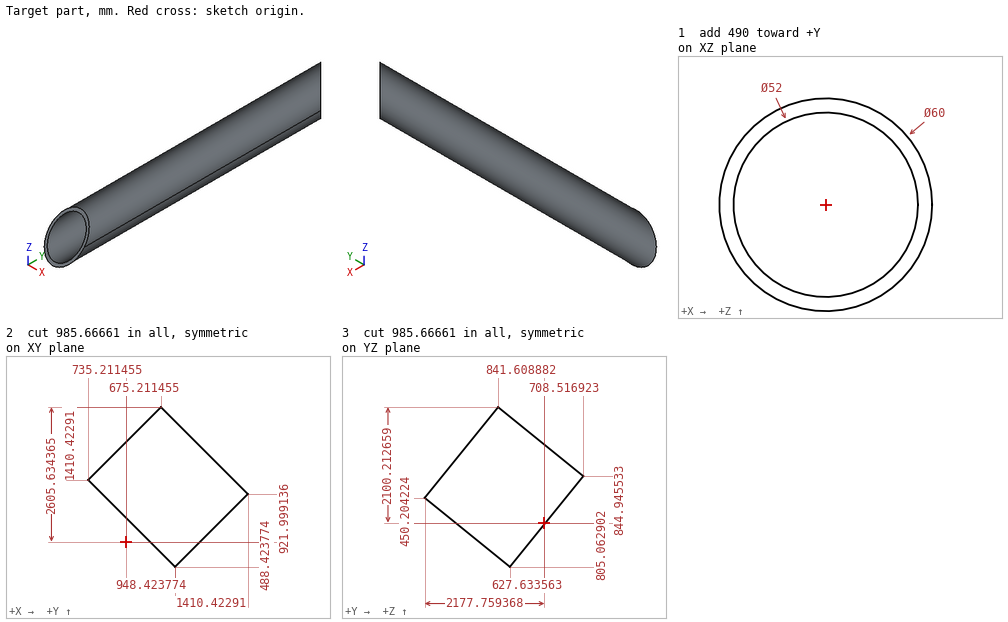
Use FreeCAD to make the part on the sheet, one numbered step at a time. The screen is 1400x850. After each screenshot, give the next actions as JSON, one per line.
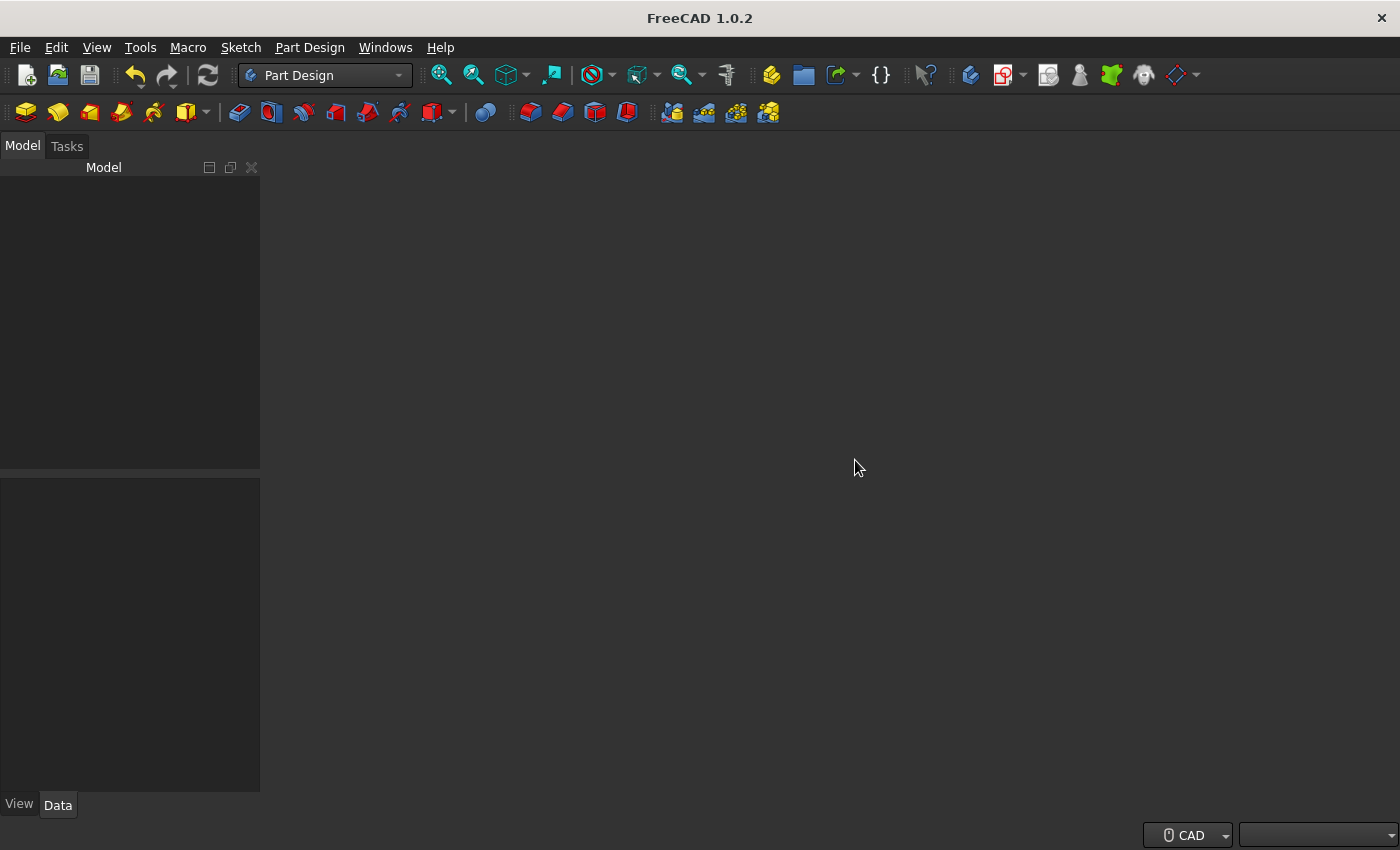
{"action": "key", "text": "ctrl+n"}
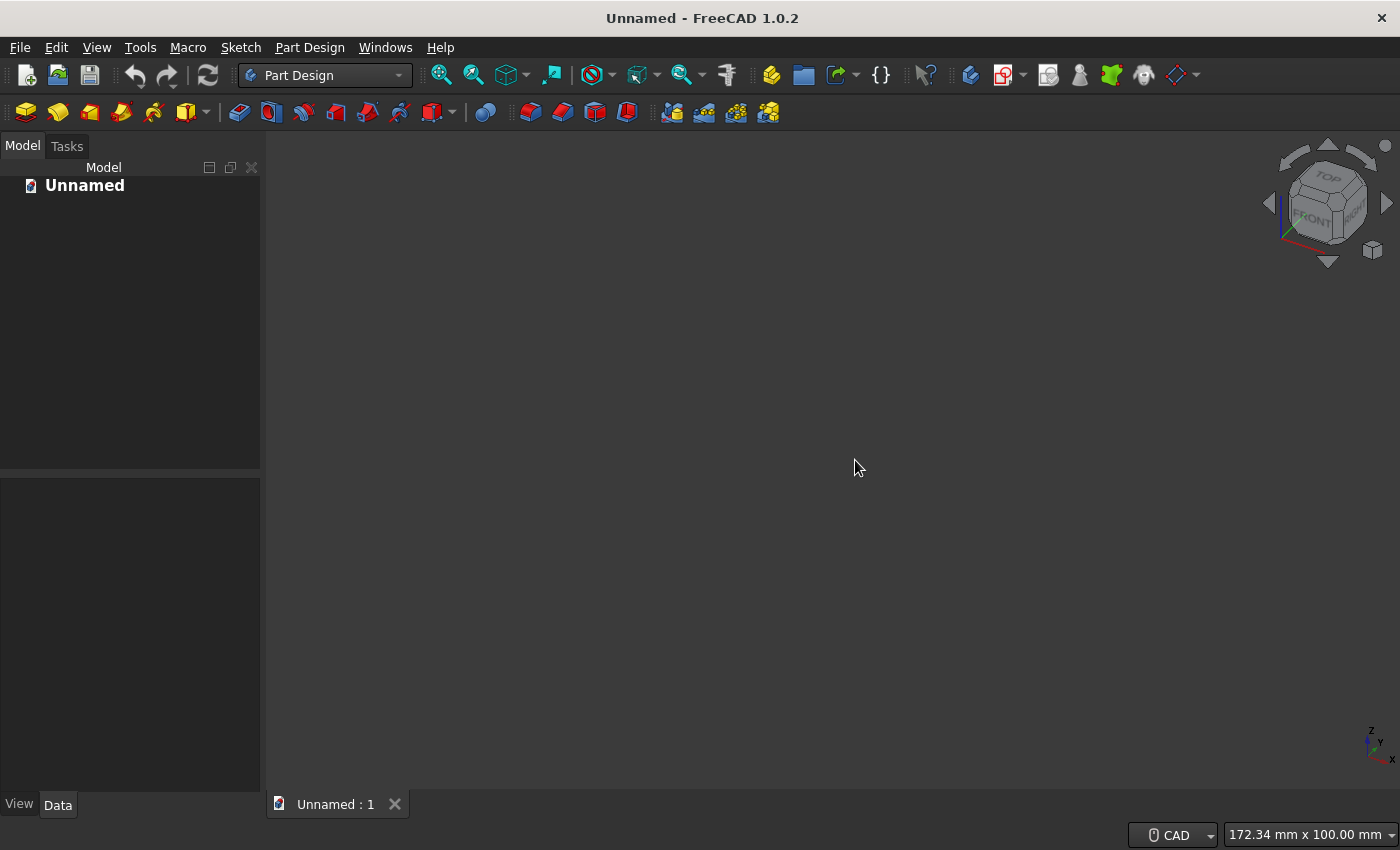
{"action": "left_click", "coordinate": [1004, 76]}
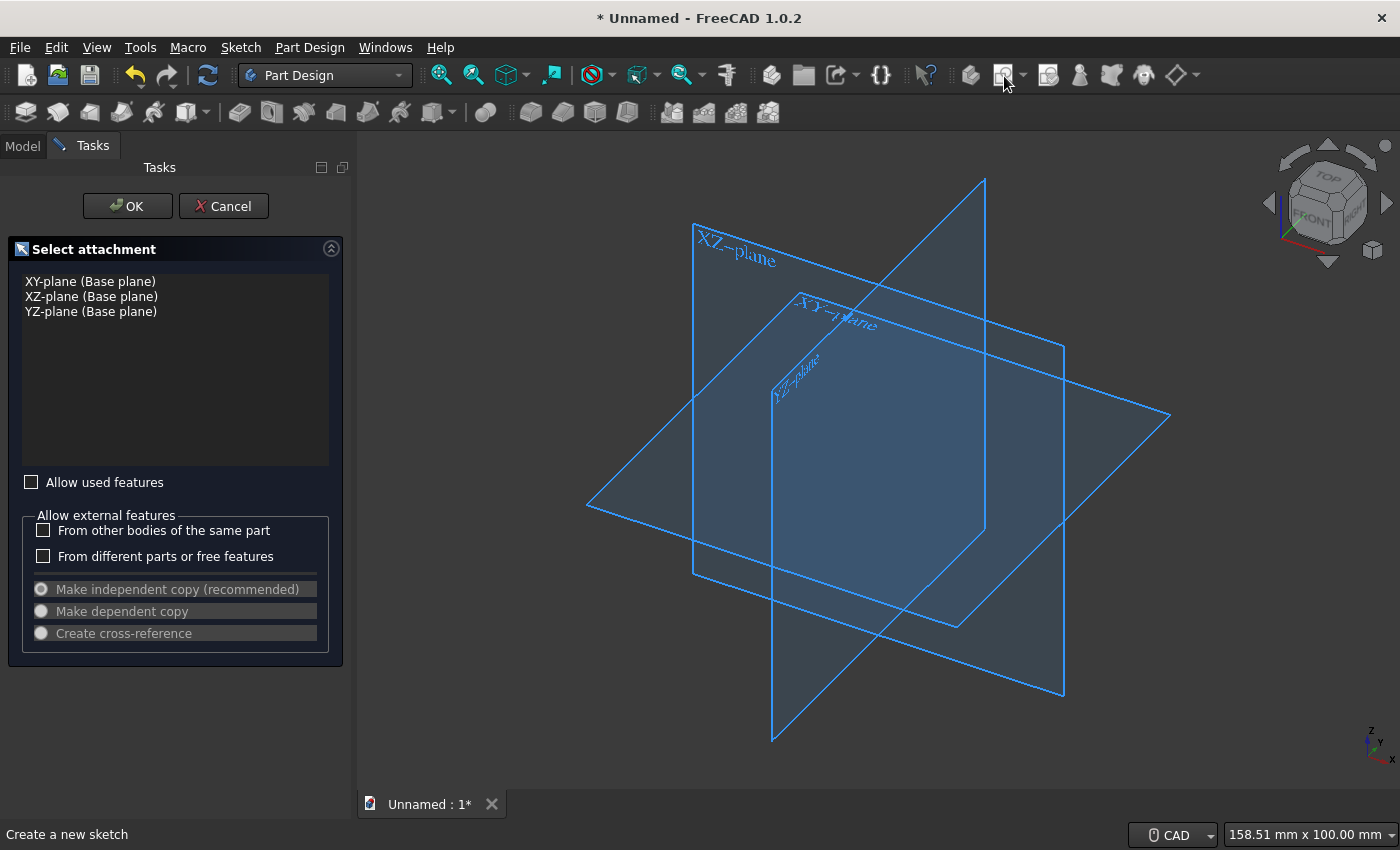
{"action": "left_click", "coordinate": [82, 296]}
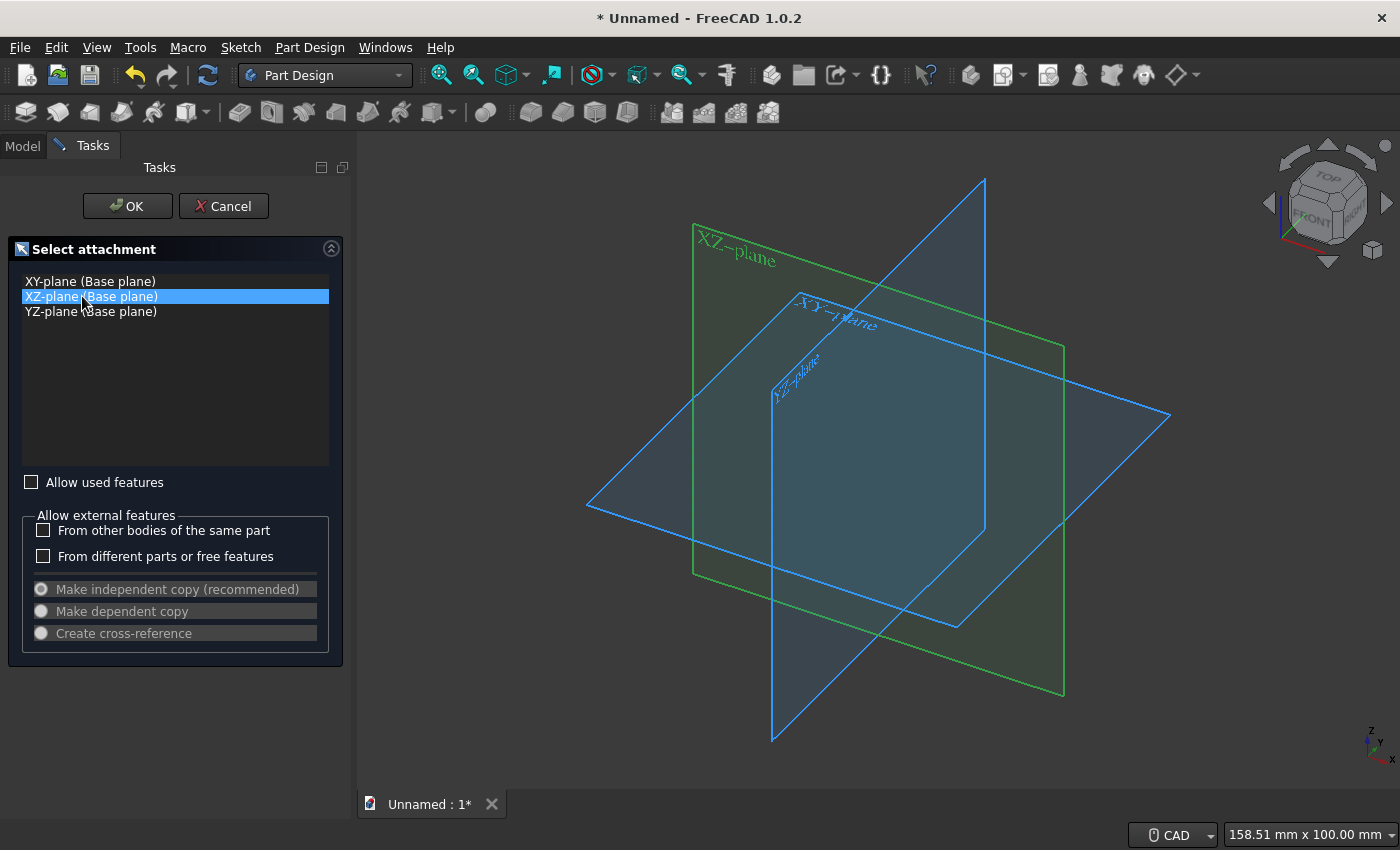
{"action": "left_click", "coordinate": [128, 206]}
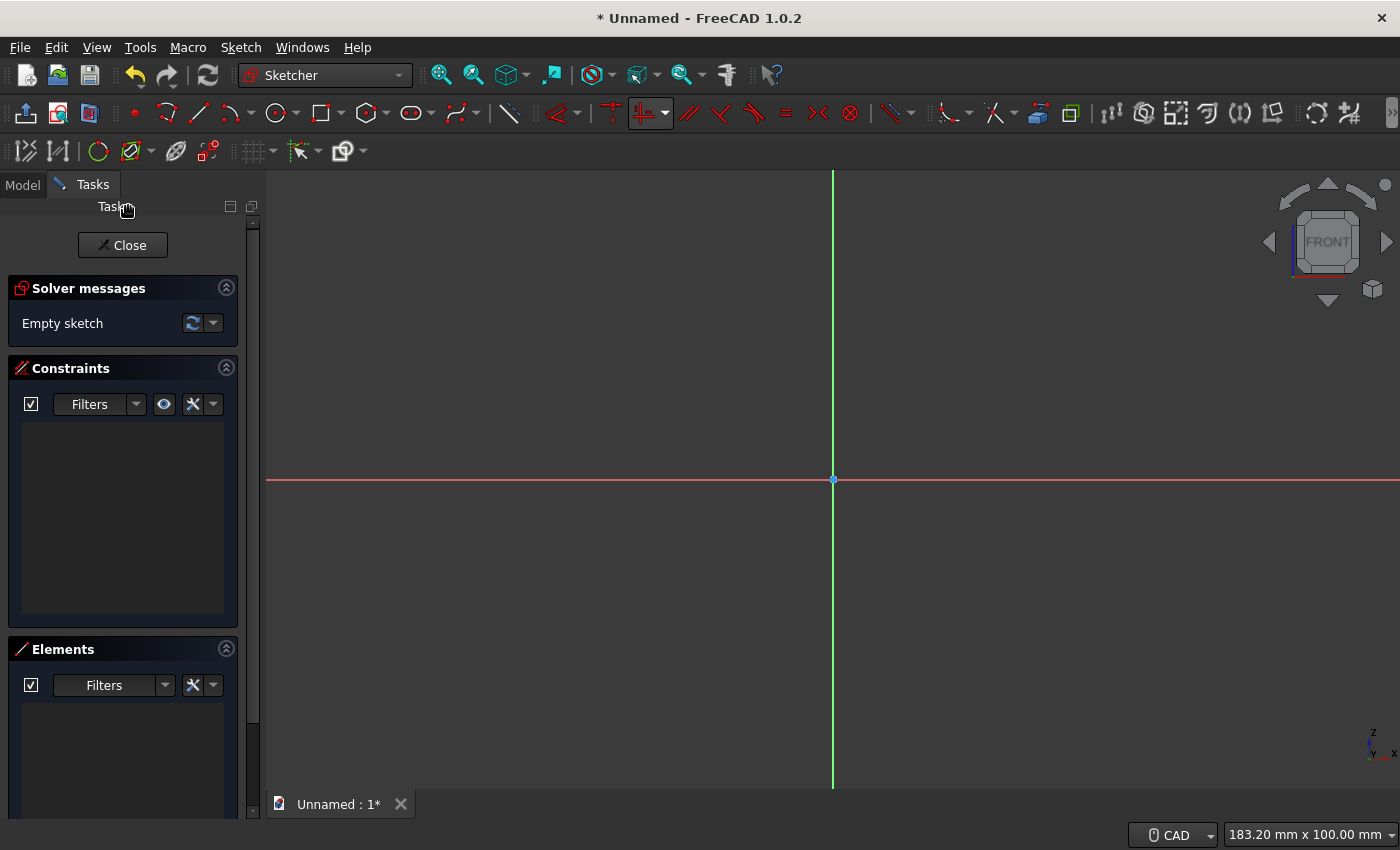
{"action": "key", "text": "g c"}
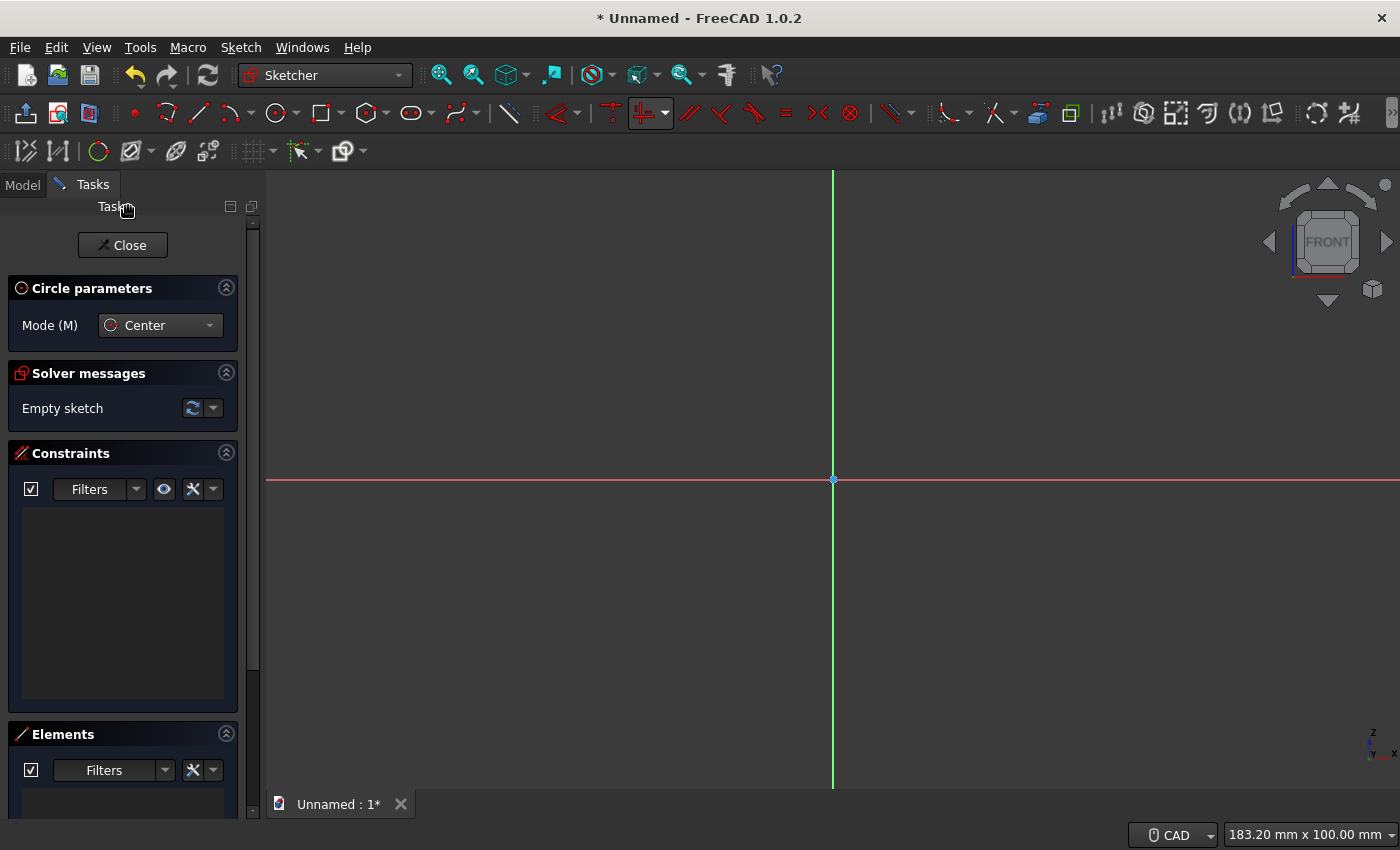
{"action": "left_click", "coordinate": [833, 480]}
{"action": "mouse_move", "coordinate": [964, 348]}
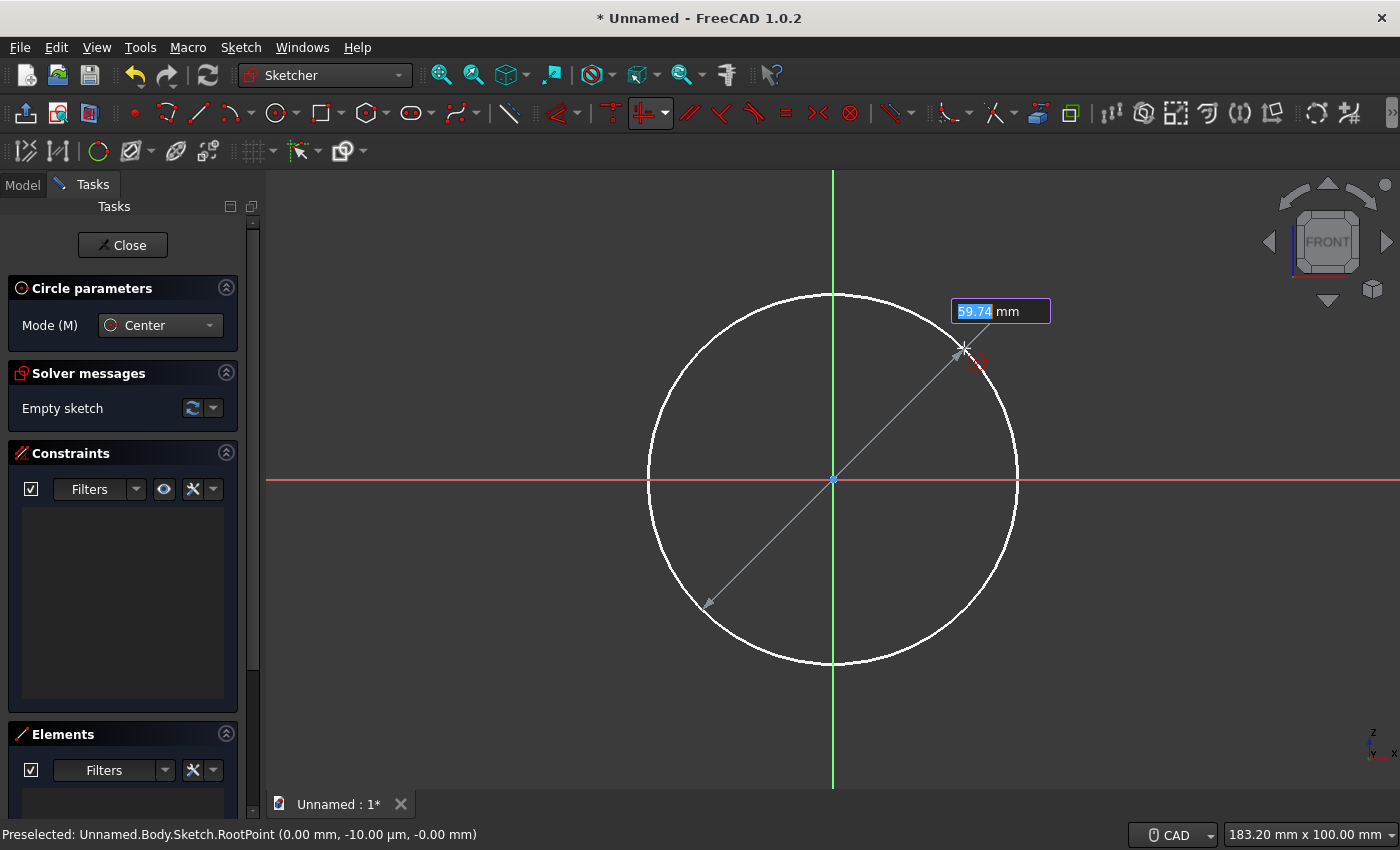
{"action": "type", "text": "60"}
{"action": "key", "text": "Return"}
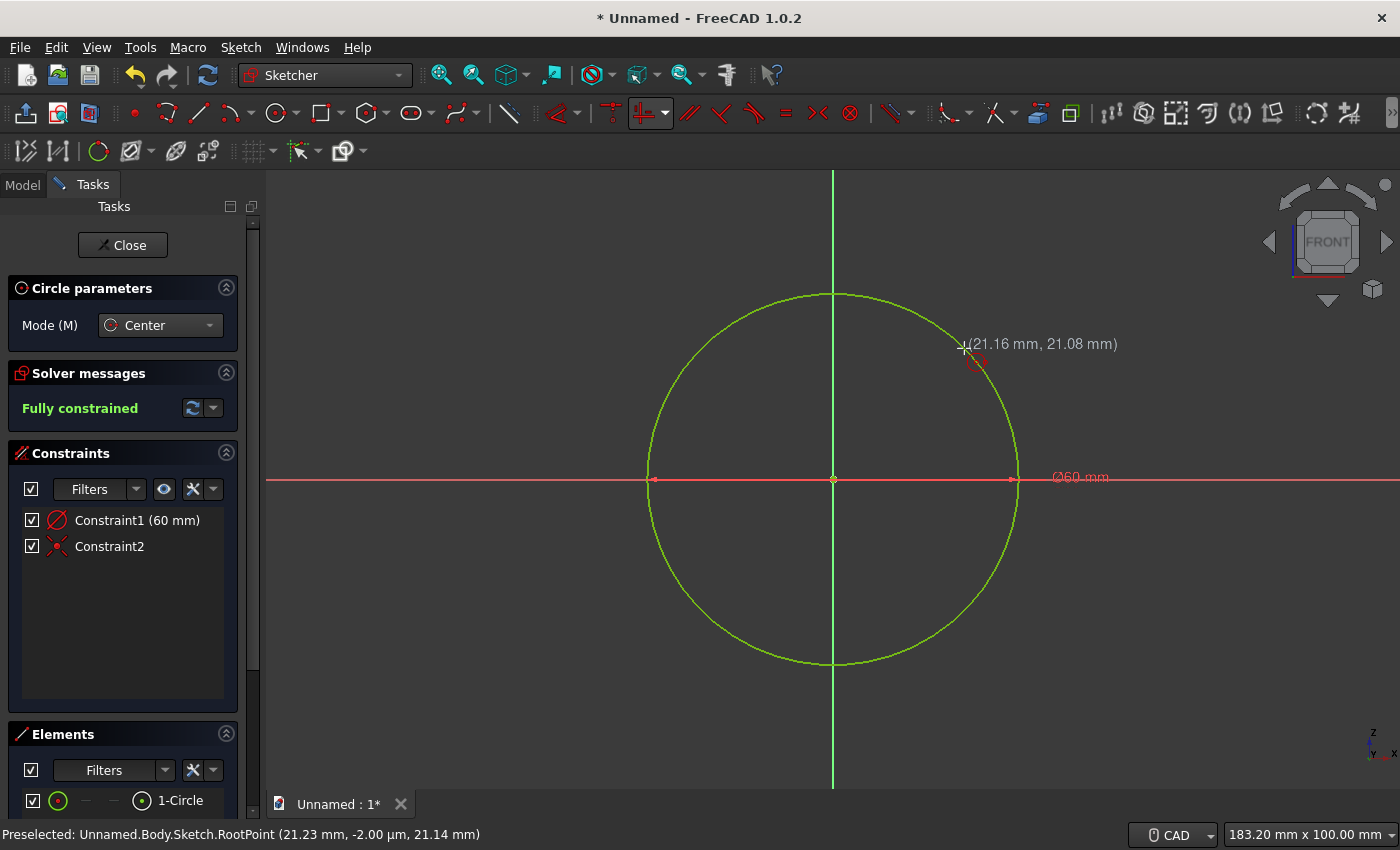
{"action": "left_click", "coordinate": [833, 480]}
{"action": "mouse_move", "coordinate": [947, 366]}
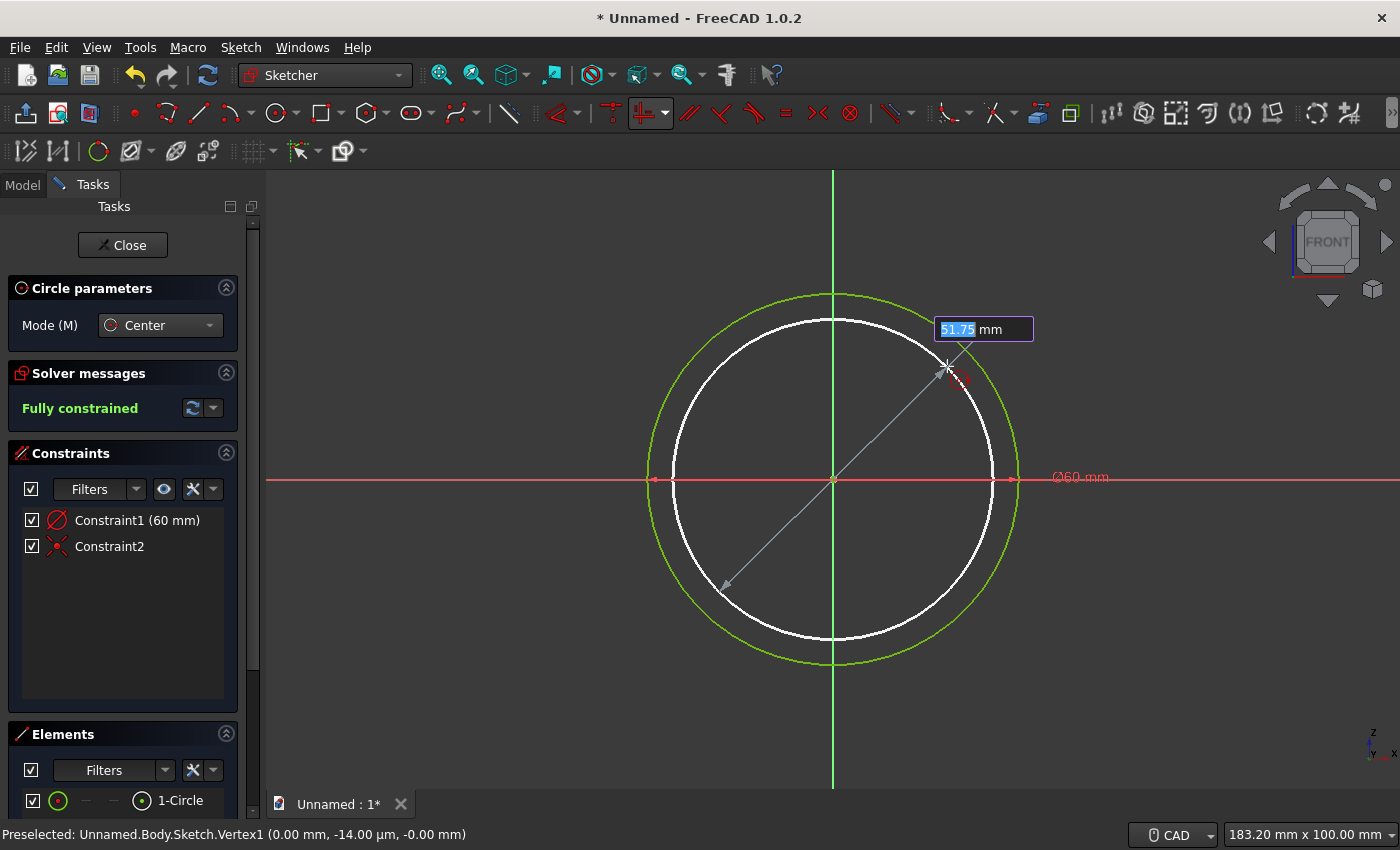
{"action": "type", "text": "52"}
{"action": "key", "text": "Return"}
{"action": "key", "text": "Escape"}